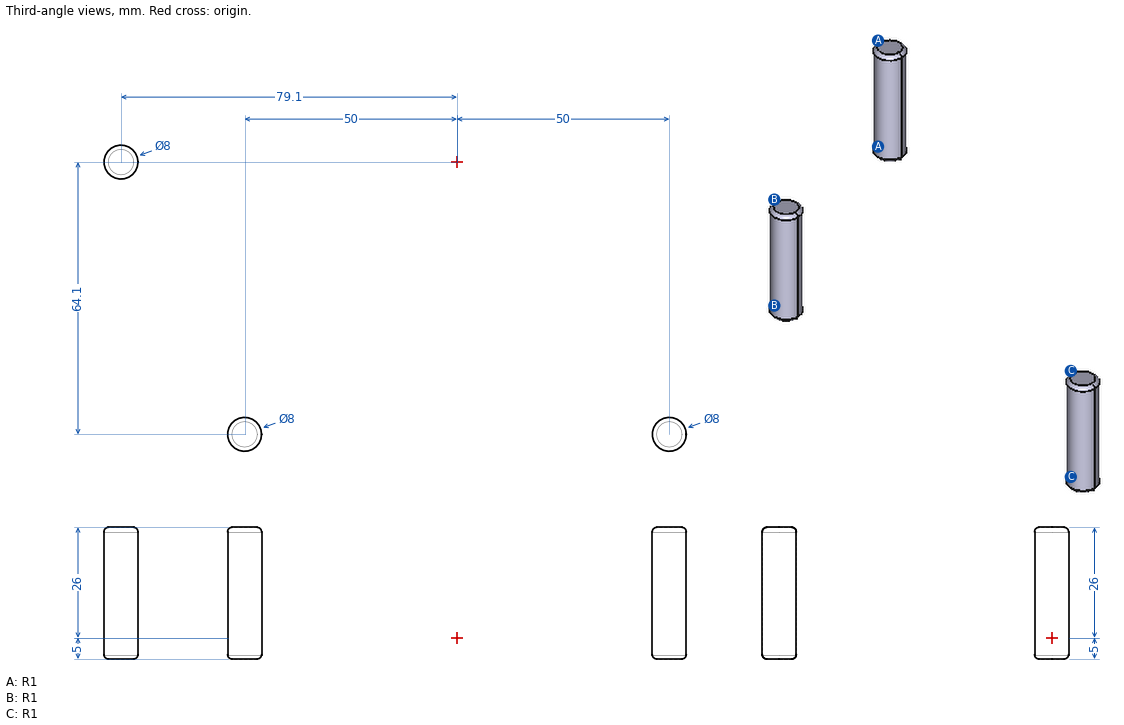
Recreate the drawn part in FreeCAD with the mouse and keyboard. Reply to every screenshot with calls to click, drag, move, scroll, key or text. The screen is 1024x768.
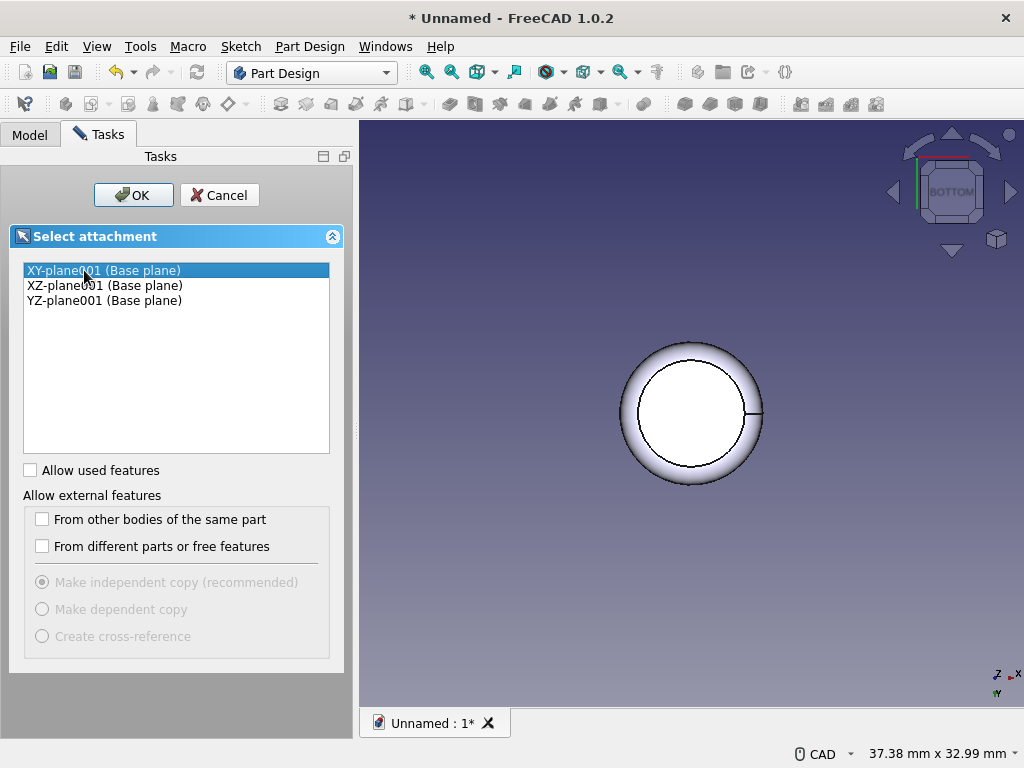
click(134, 195)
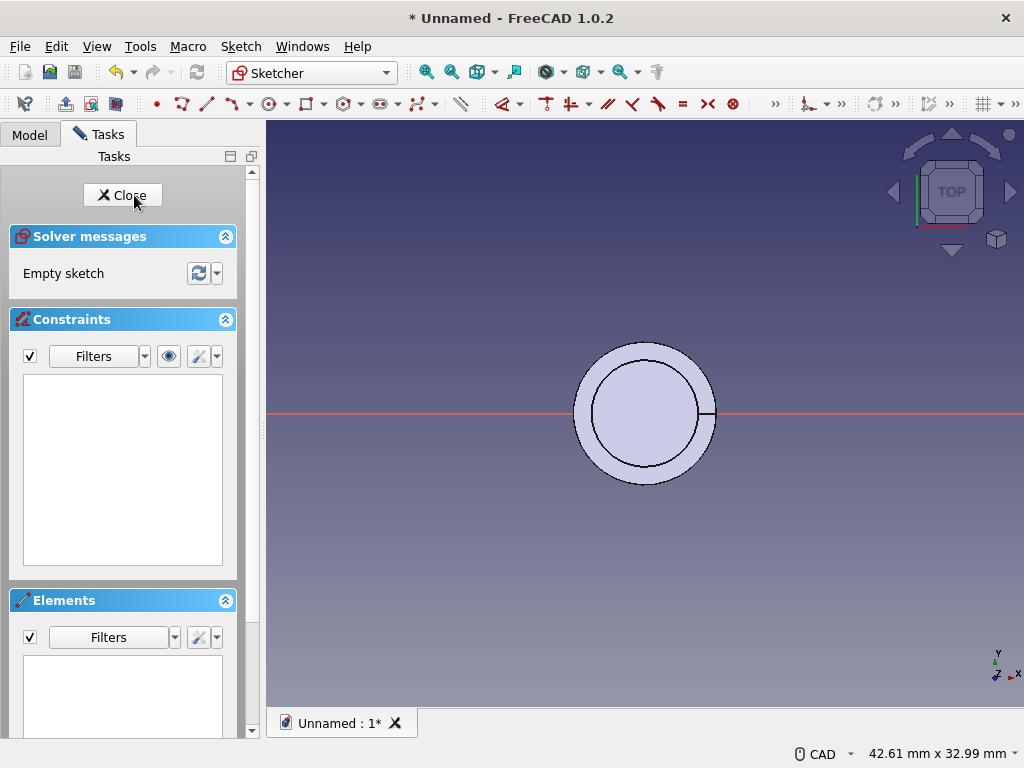
scroll(576, 414, down, 5)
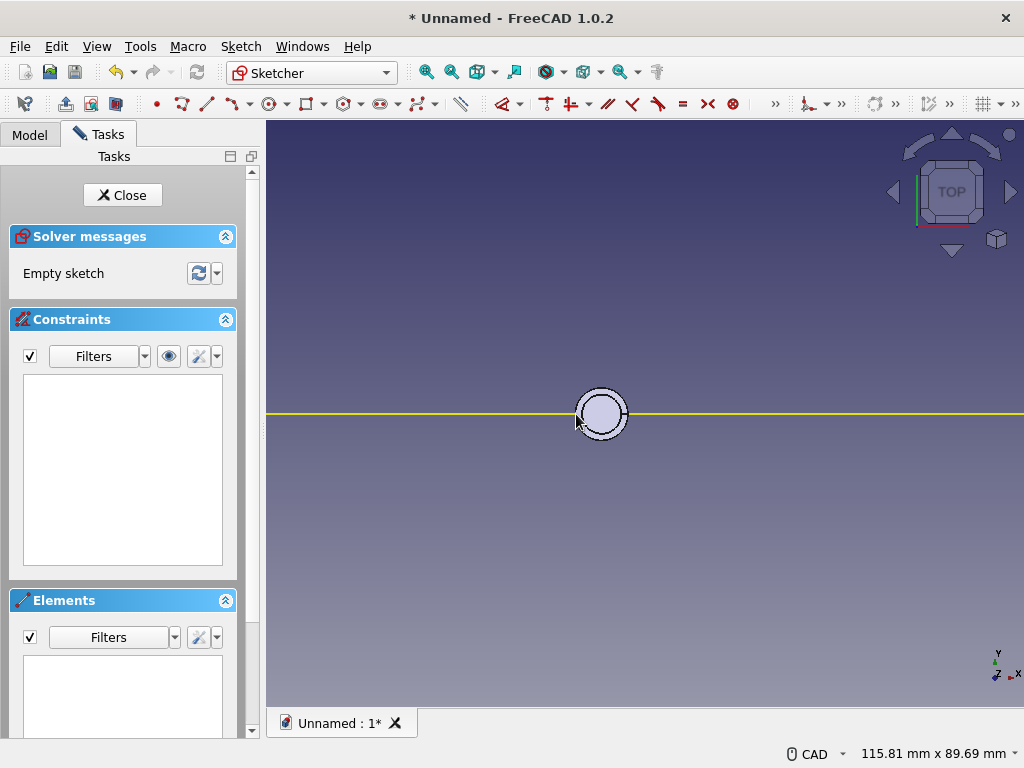
scroll(576, 414, down, 5)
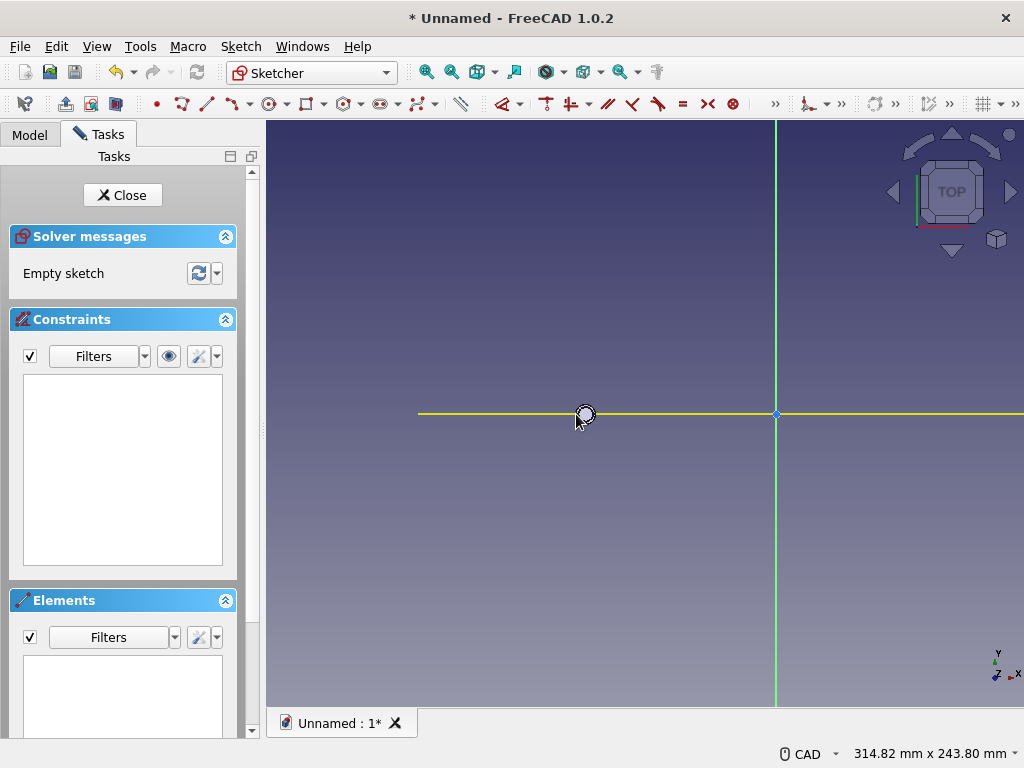
scroll(660, 577, up, 15)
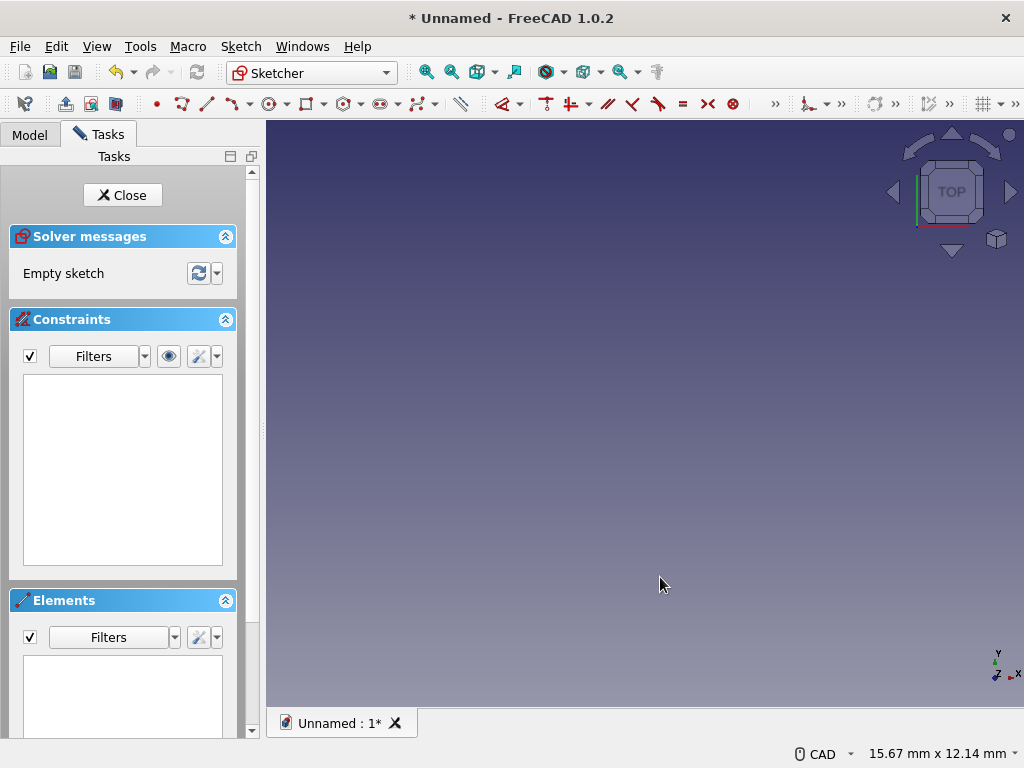
click(268, 104)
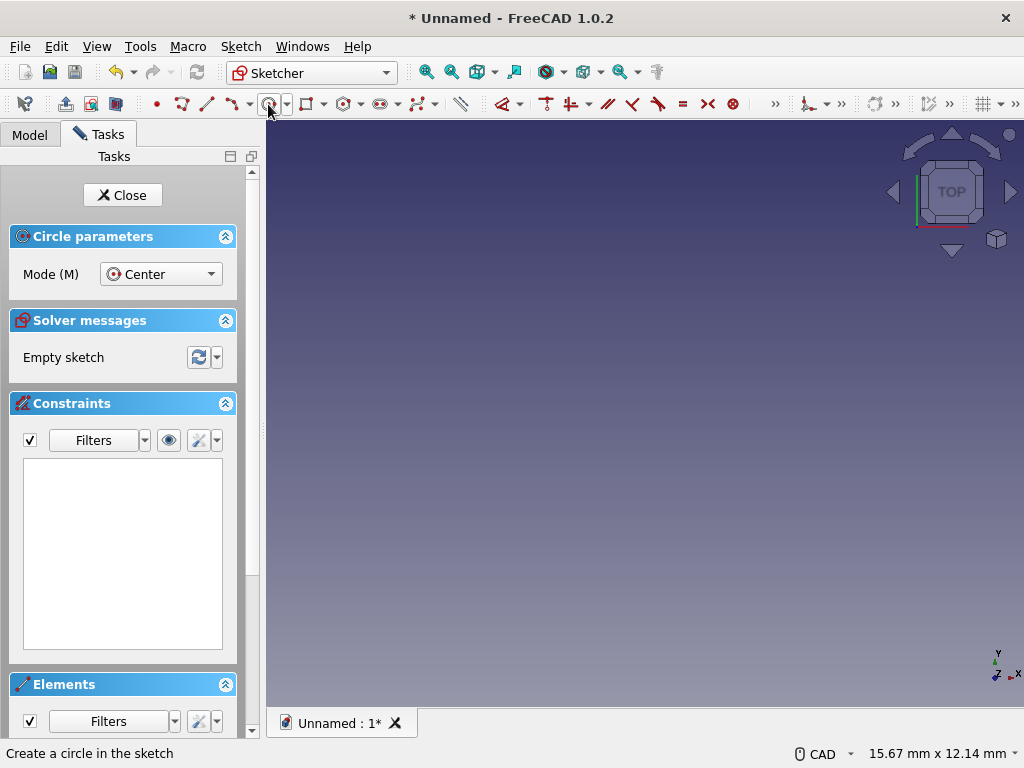
click(564, 395)
click(701, 259)
key(Escape)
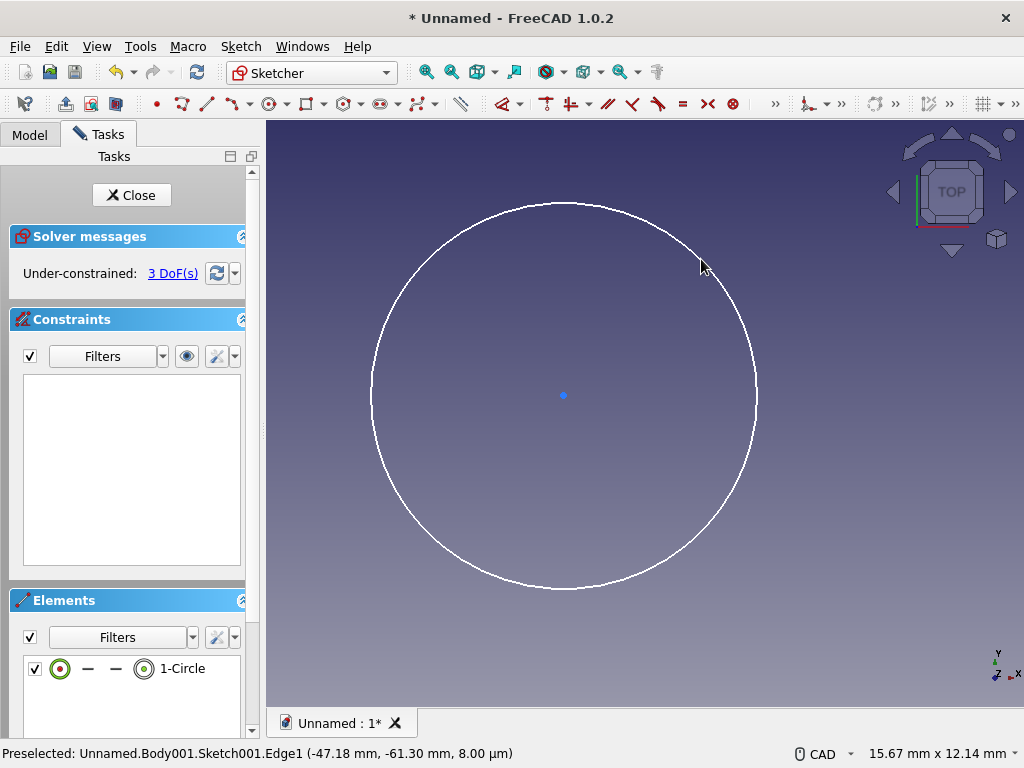
click(502, 104)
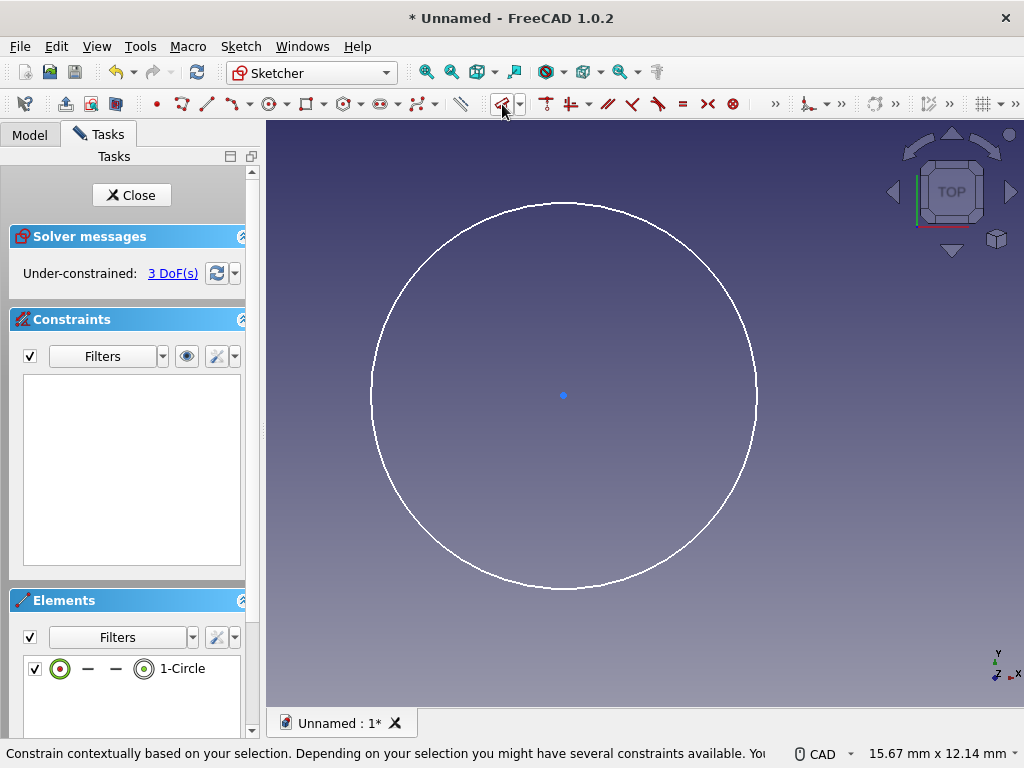
click(700, 259)
click(723, 236)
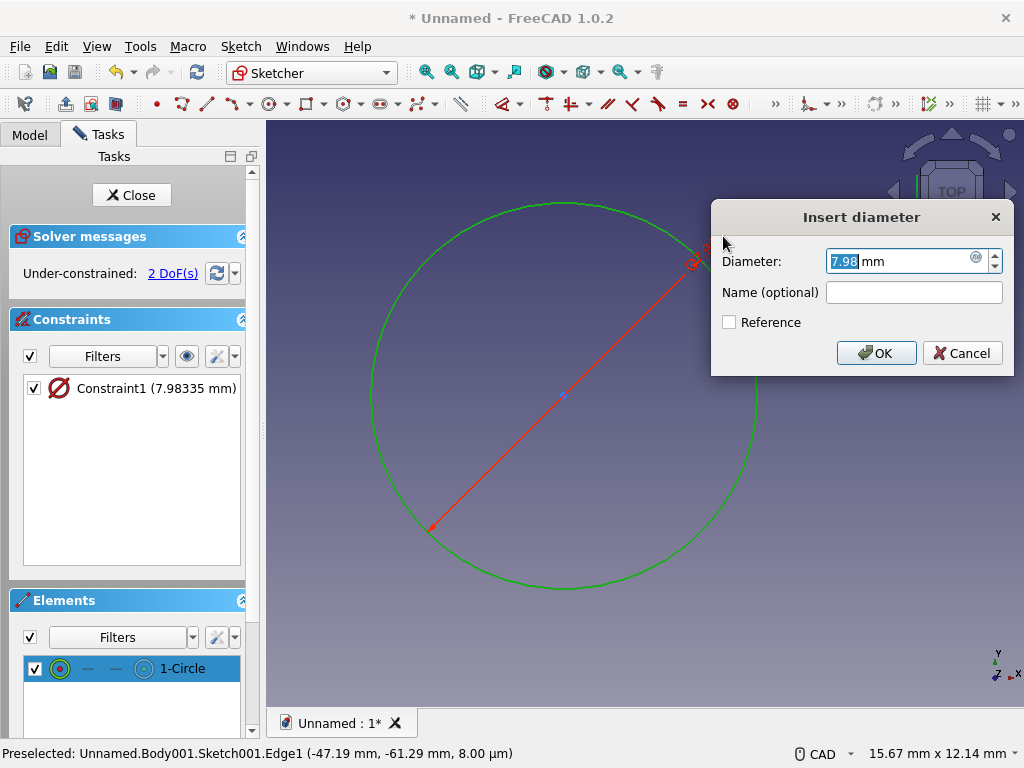
text(8)
key(Return)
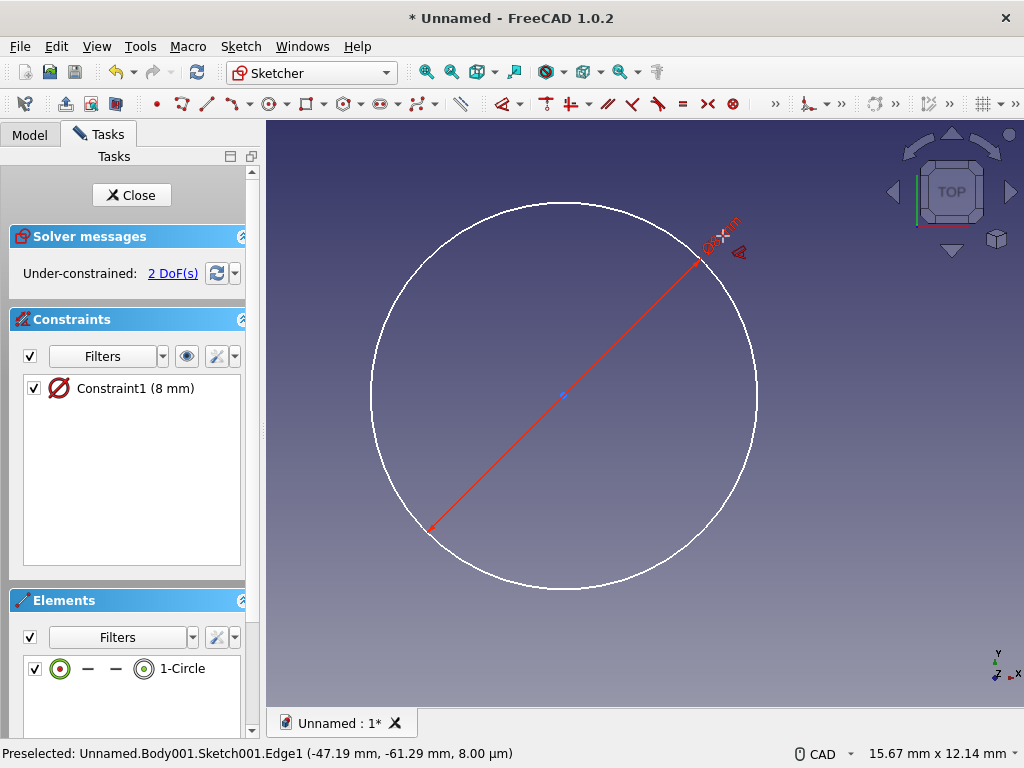
click(564, 396)
click(711, 430)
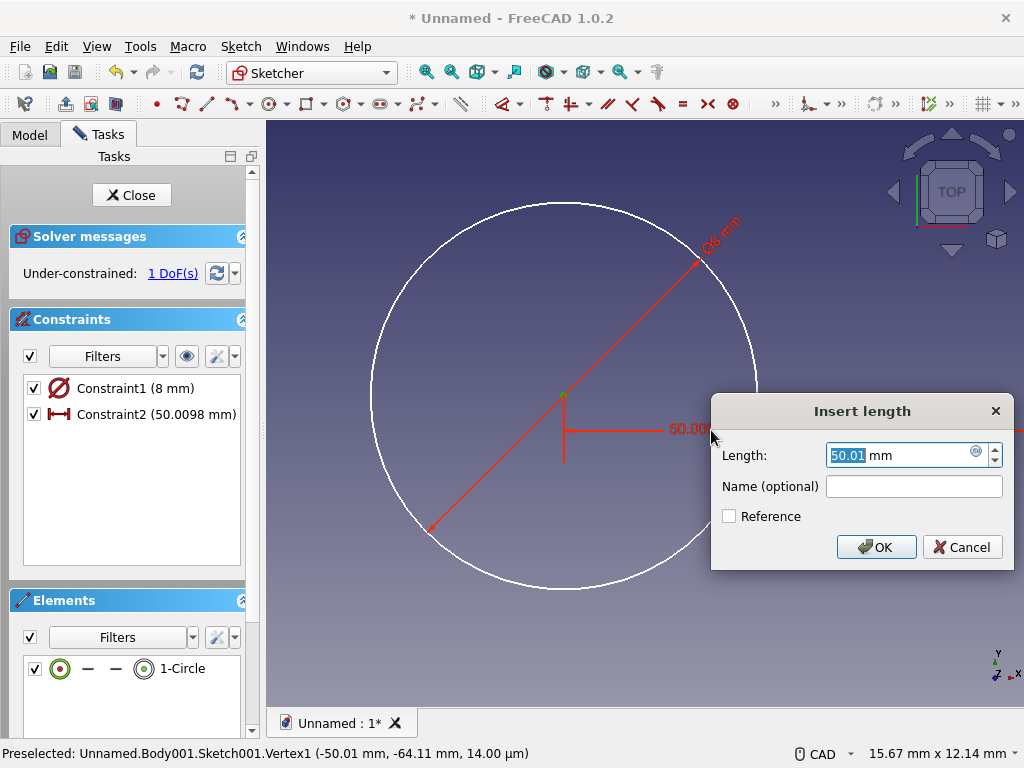
text(50)
key(Return)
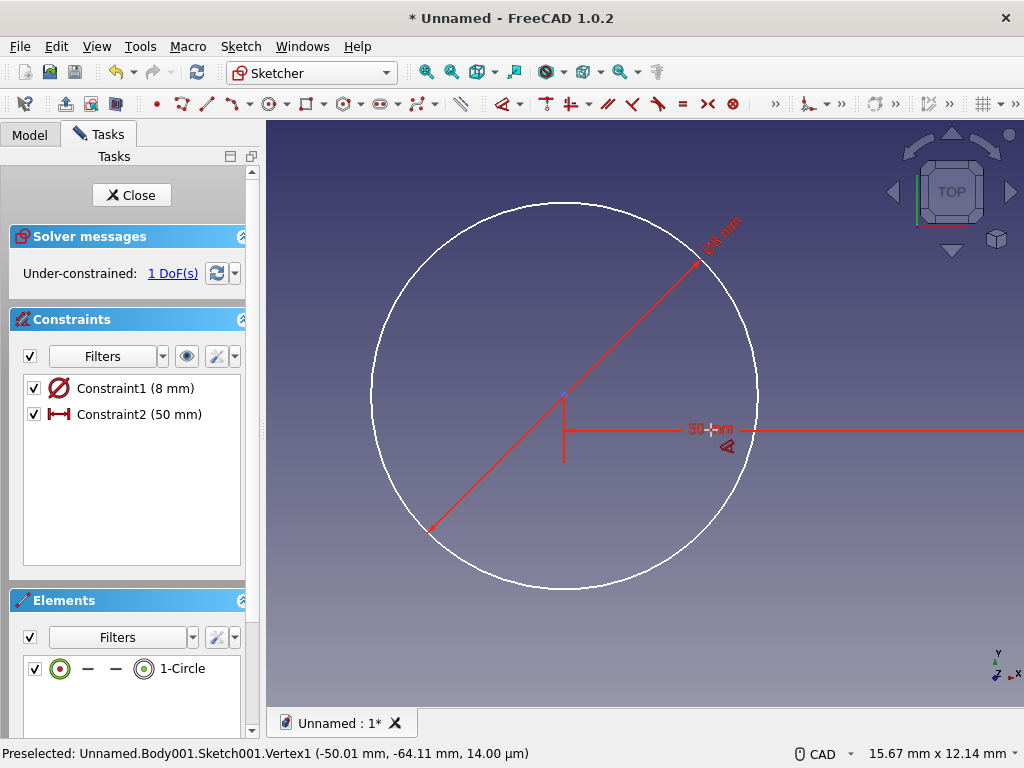
click(564, 396)
click(530, 272)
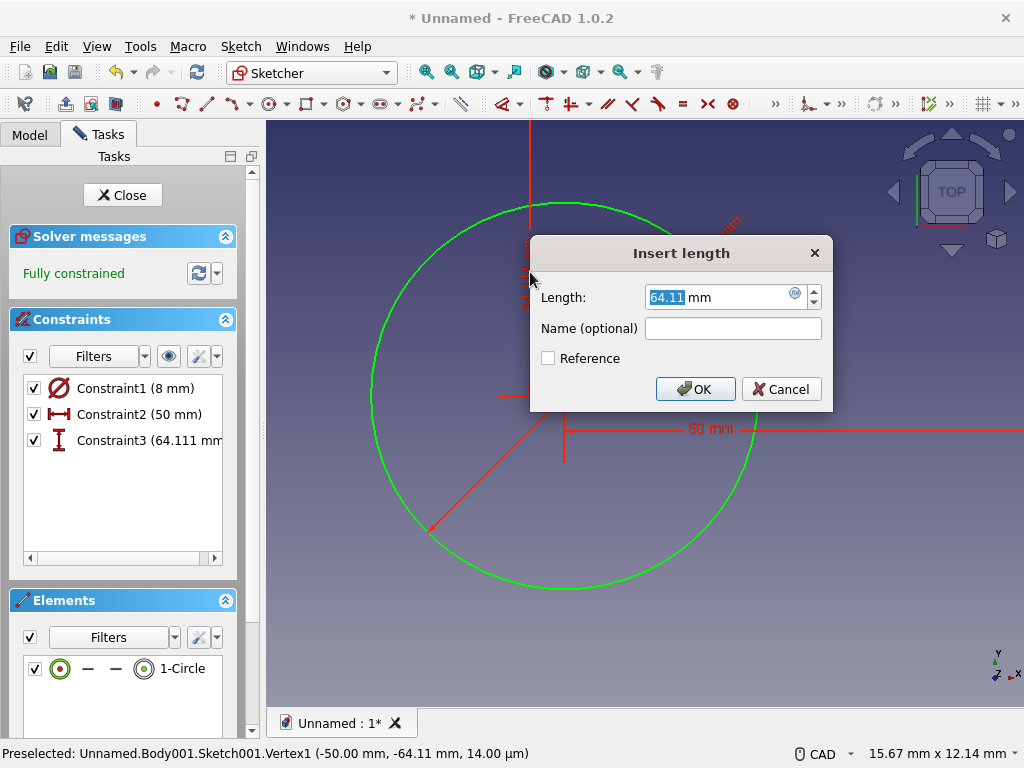
text(64.1)
key(Return)
key(Escape)